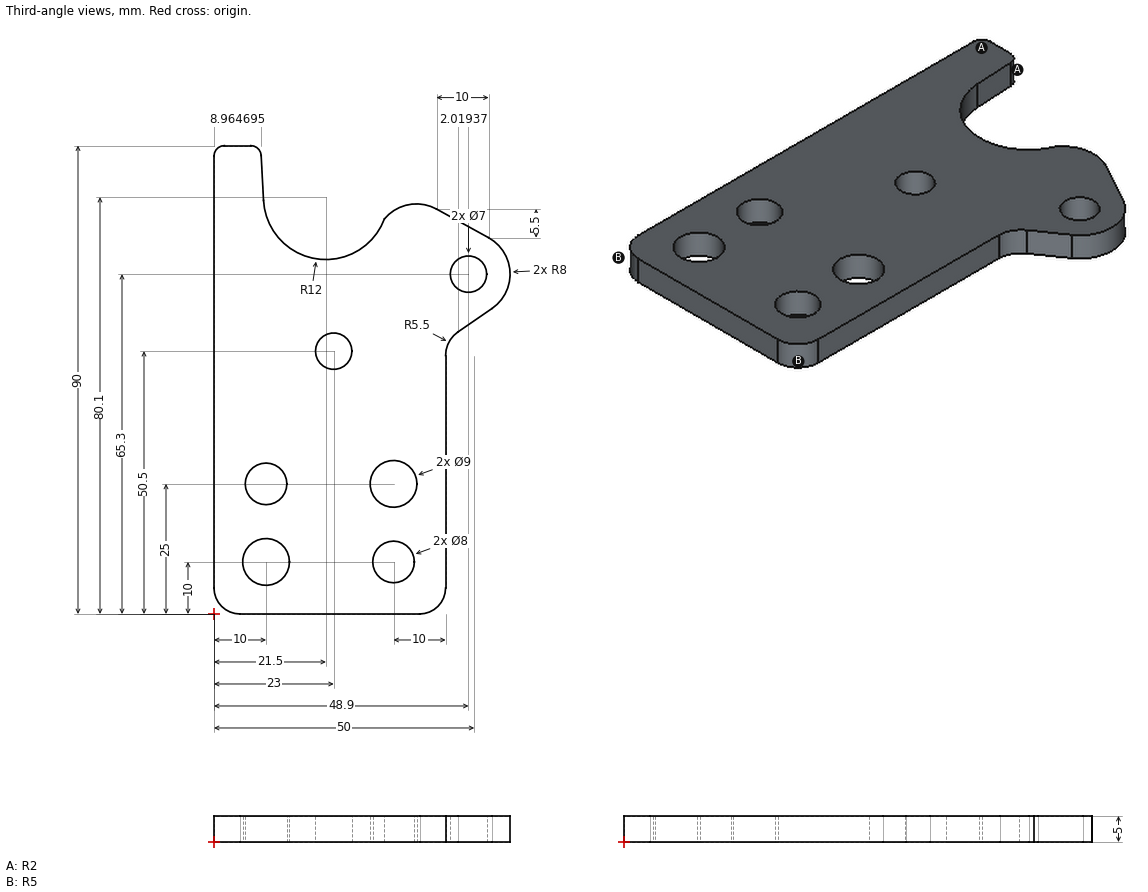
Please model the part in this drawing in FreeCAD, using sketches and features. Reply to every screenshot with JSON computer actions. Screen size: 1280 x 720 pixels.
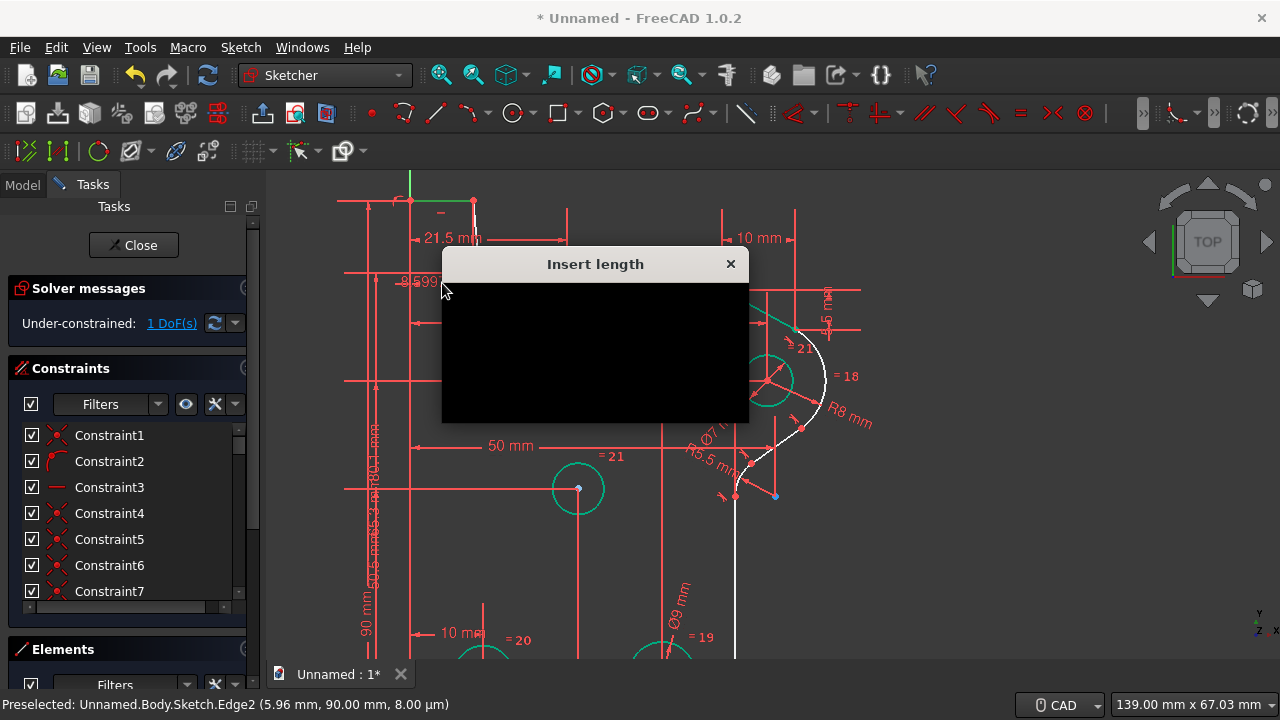
{"action": "type", "text": "8.964695"}
{"action": "key", "text": "Return"}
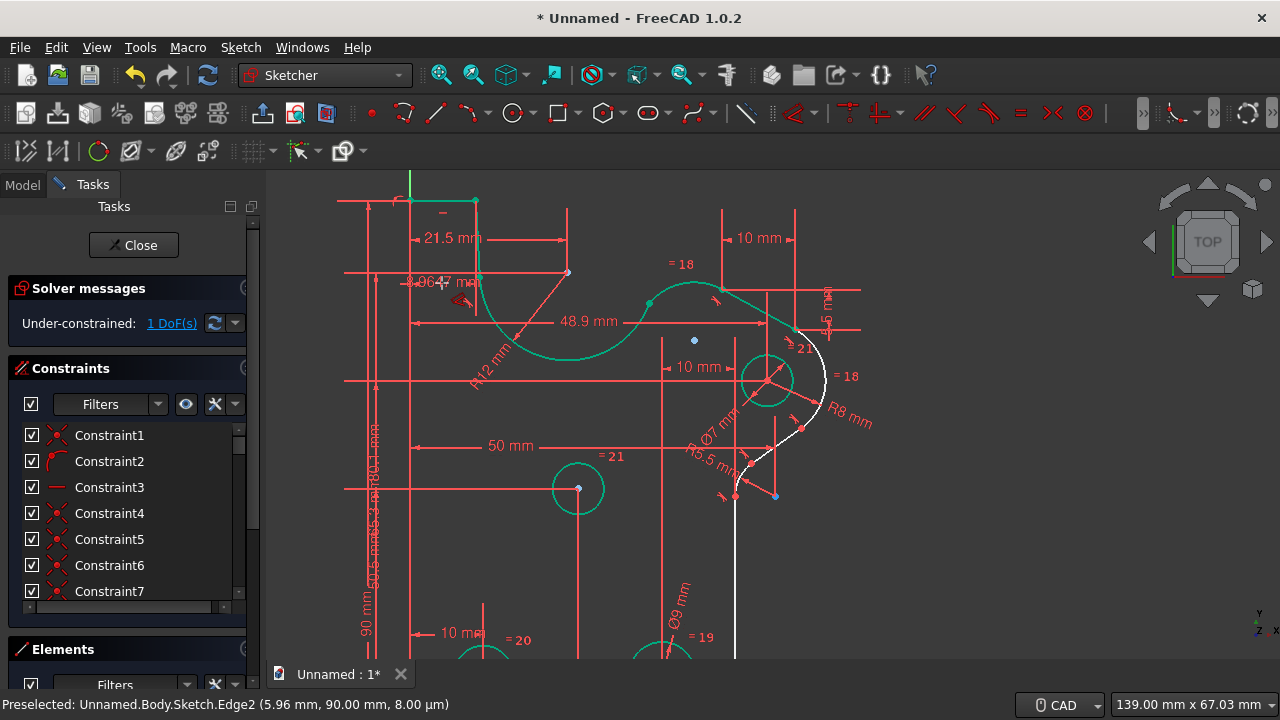
{"action": "scroll", "coordinate": [752, 464], "scroll_direction": "up", "scroll_amount": 5}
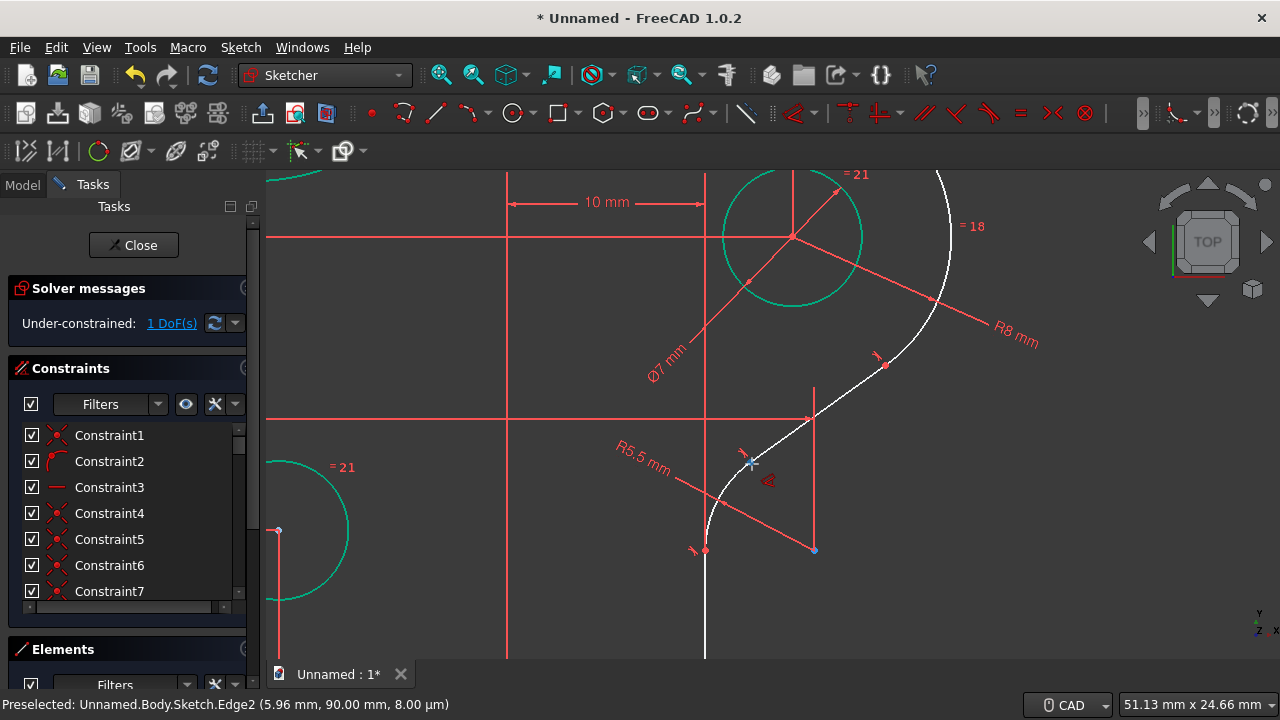
{"action": "left_click", "coordinate": [751, 462]}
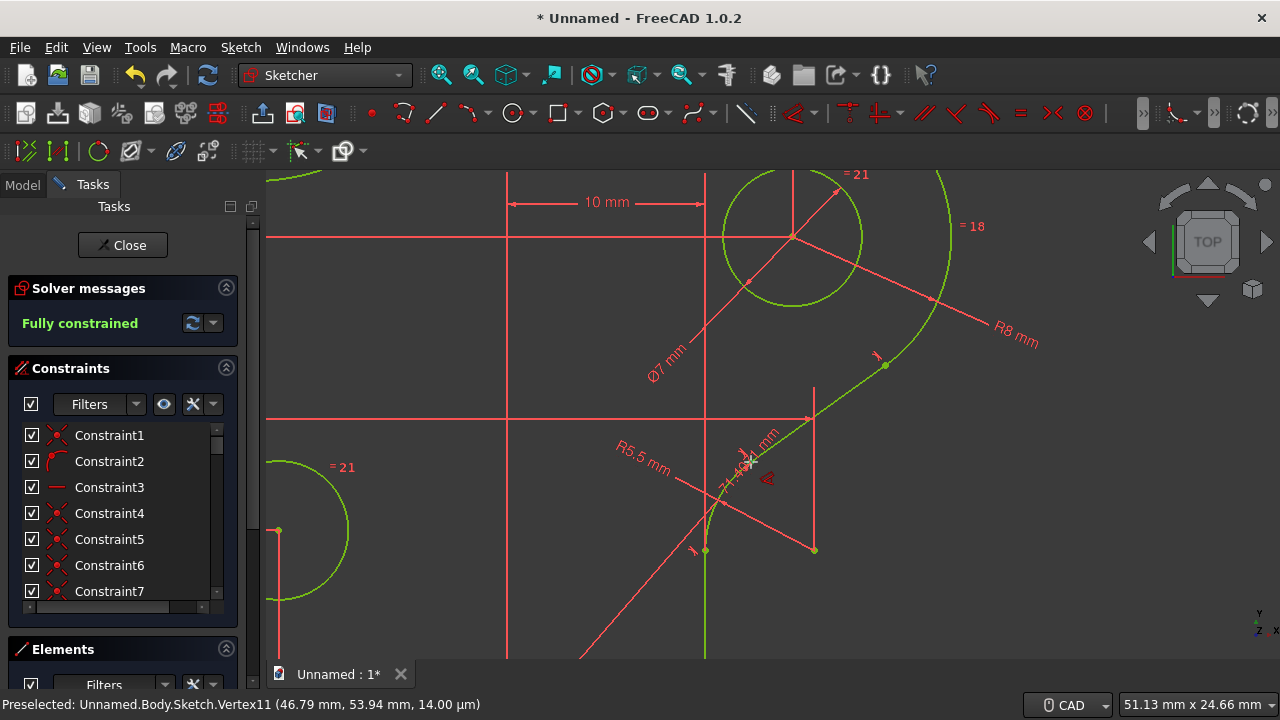
{"action": "left_click", "coordinate": [793, 237]}
{"action": "left_click", "coordinate": [772, 203]}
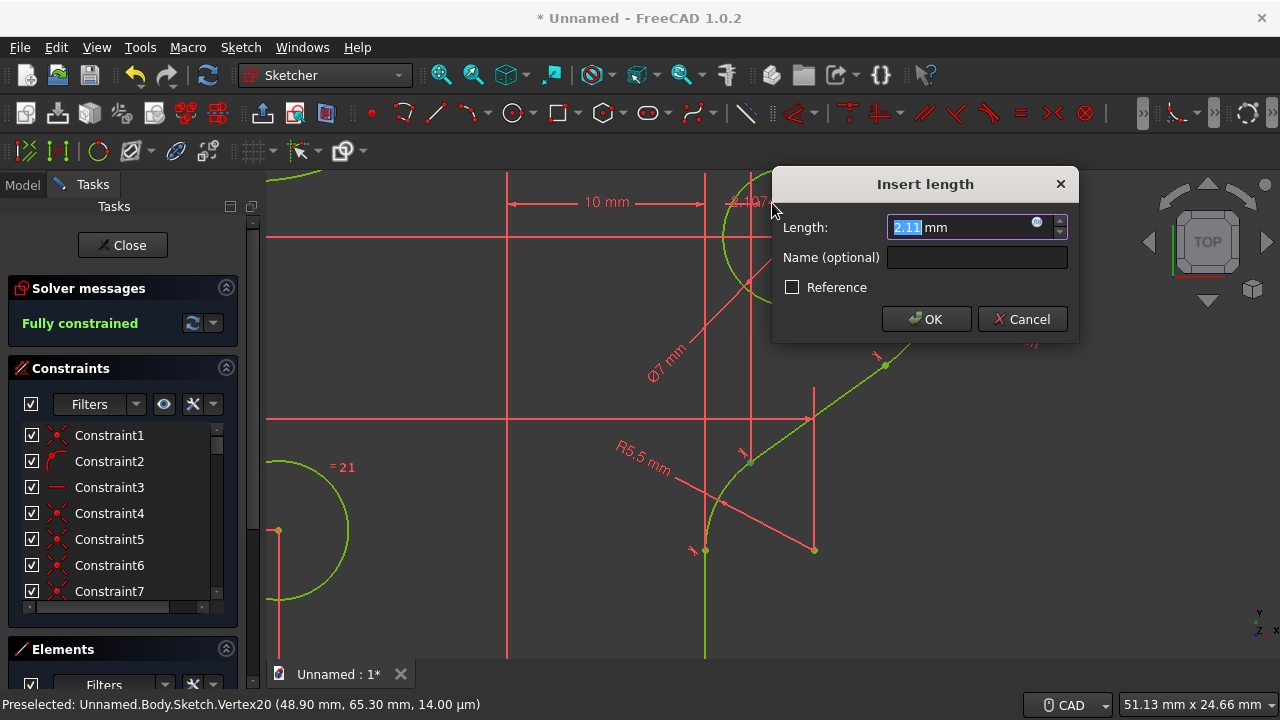
{"action": "type", "text": "2.01937"}
{"action": "key", "text": "Return"}
{"action": "key", "text": "Escape"}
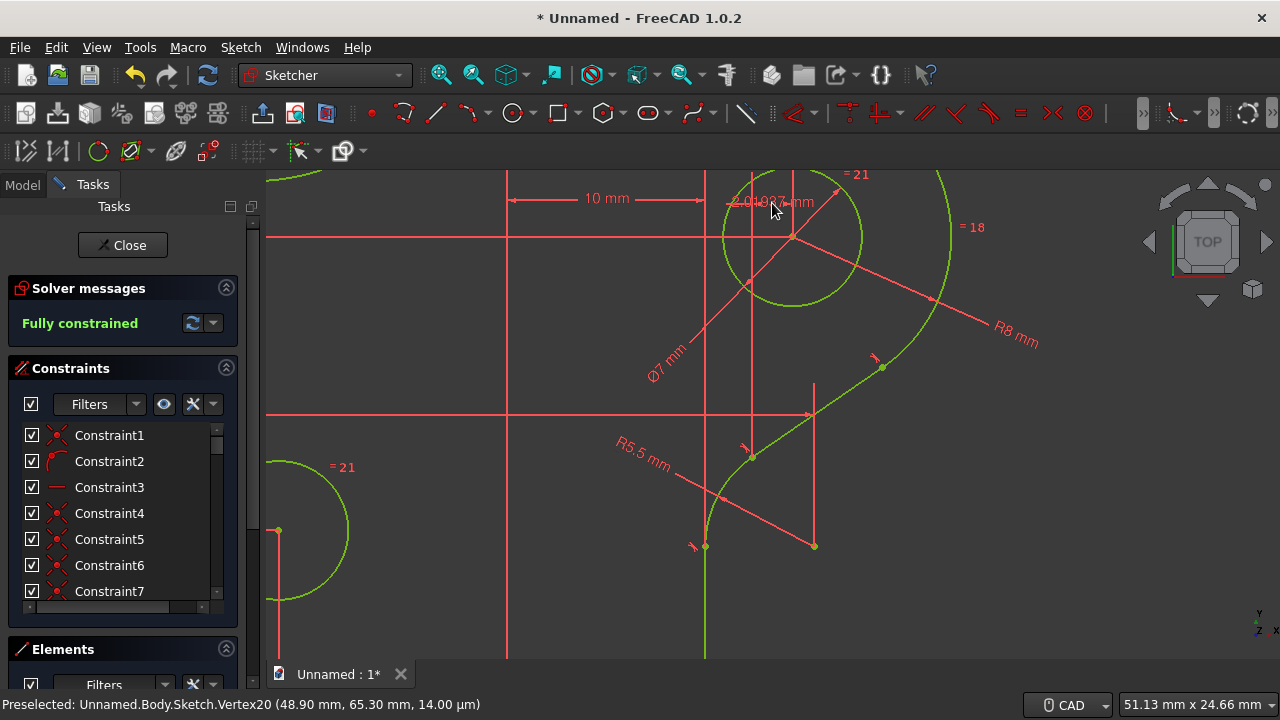
{"action": "left_click", "coordinate": [123, 245]}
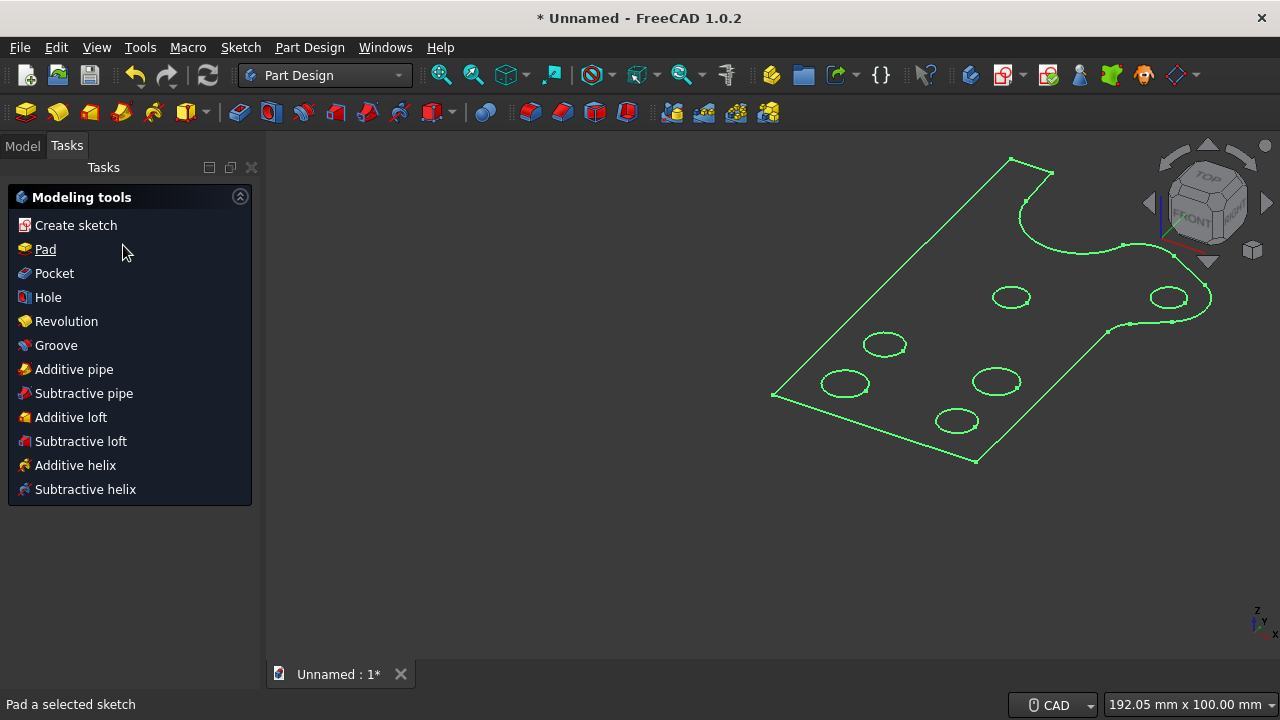
{"action": "left_click", "coordinate": [26, 112]}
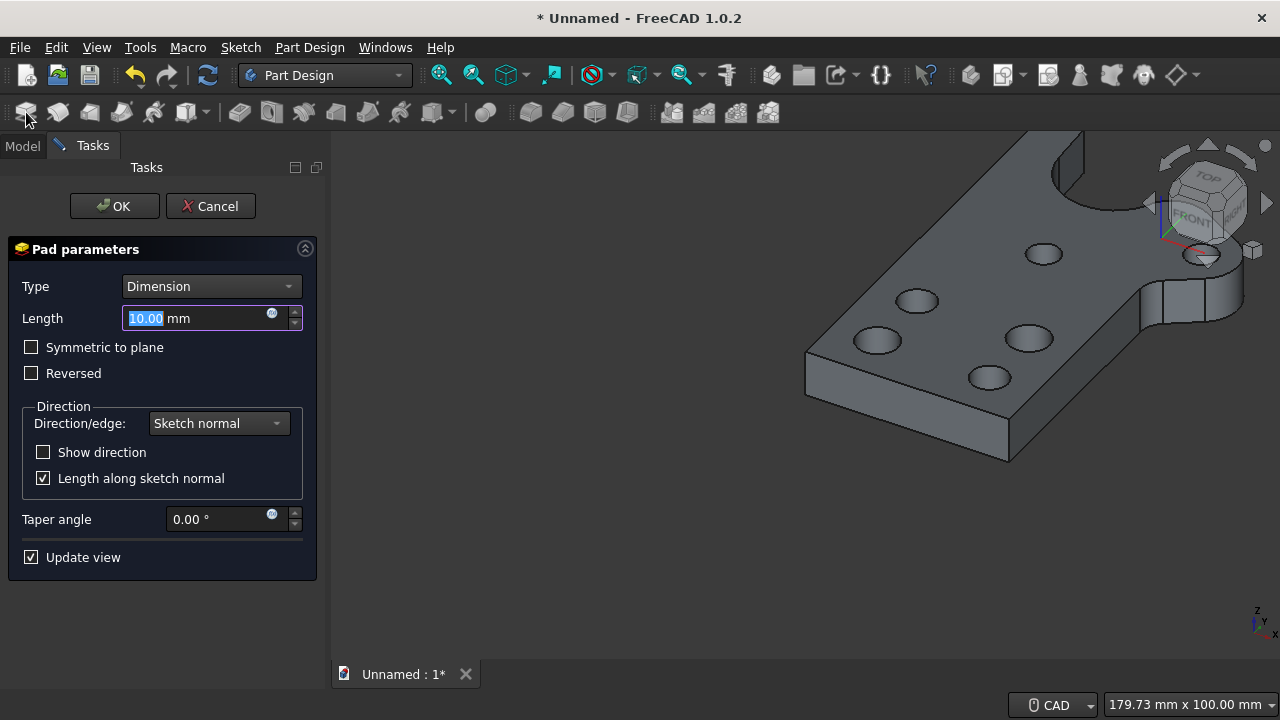
{"action": "type", "text": "5"}
{"action": "key", "text": "Tab"}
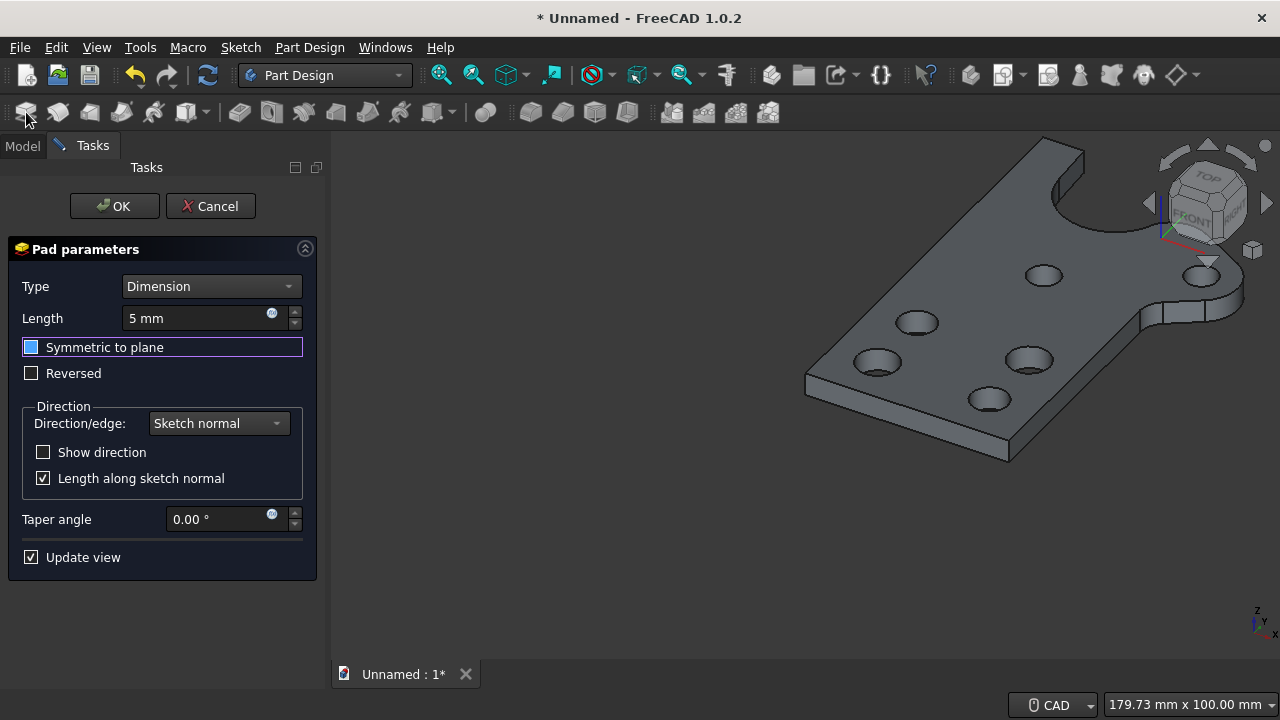
{"action": "left_click", "coordinate": [115, 206]}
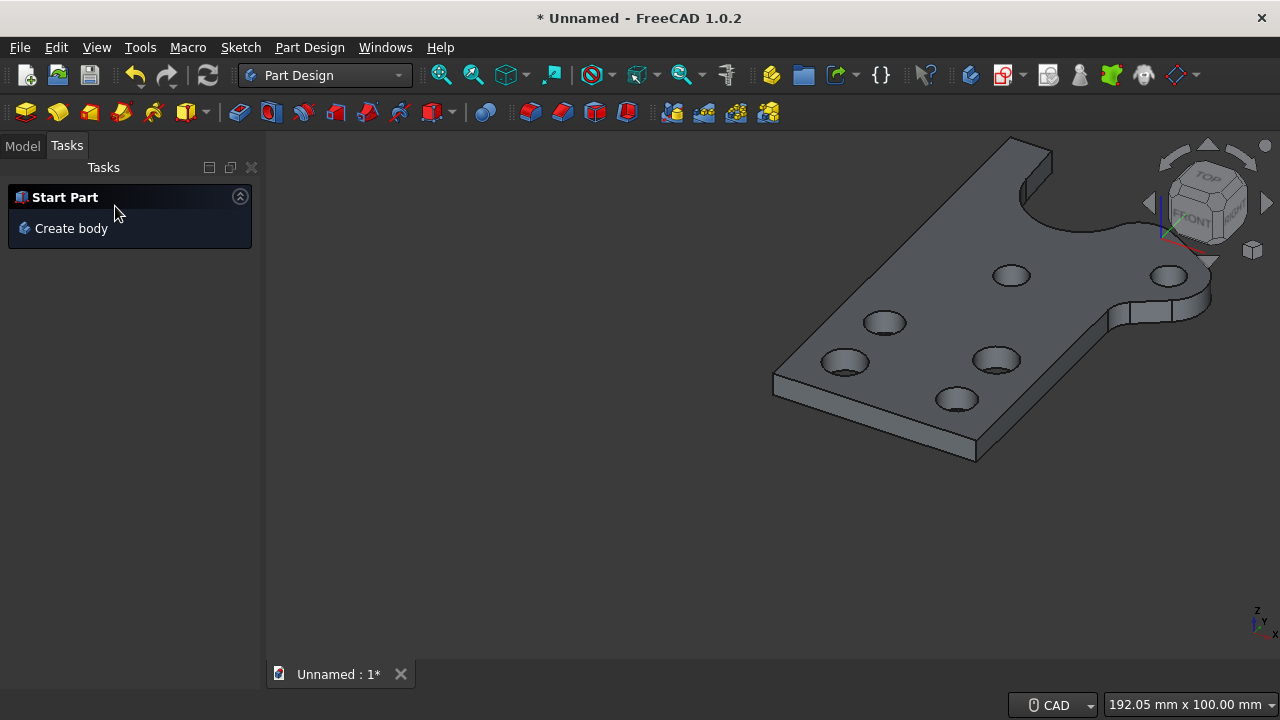
{"action": "key", "text": "0"}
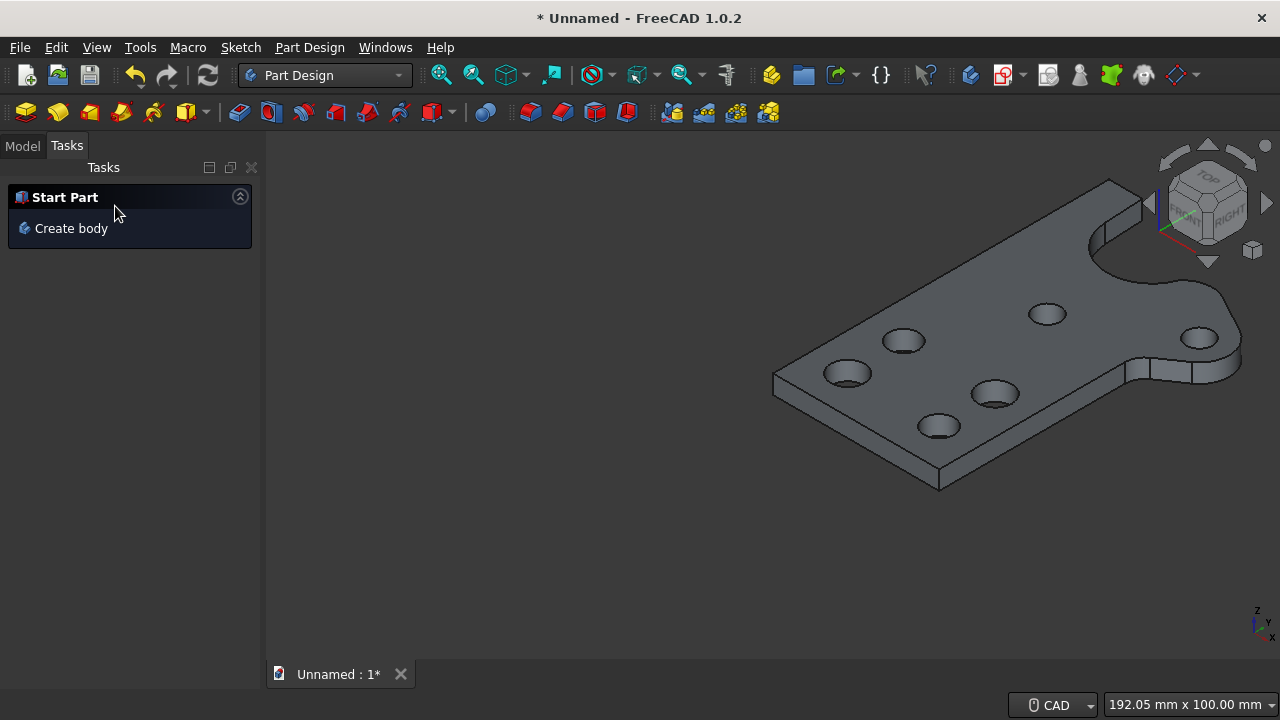
{"action": "key", "text": "v f"}